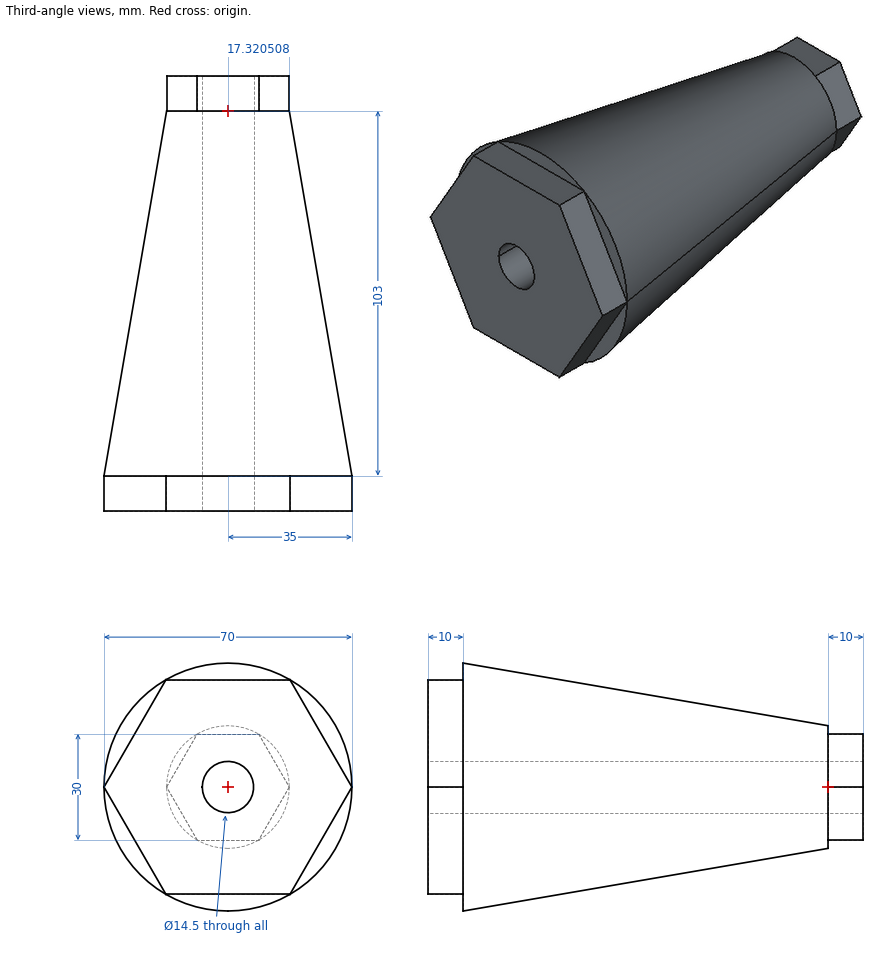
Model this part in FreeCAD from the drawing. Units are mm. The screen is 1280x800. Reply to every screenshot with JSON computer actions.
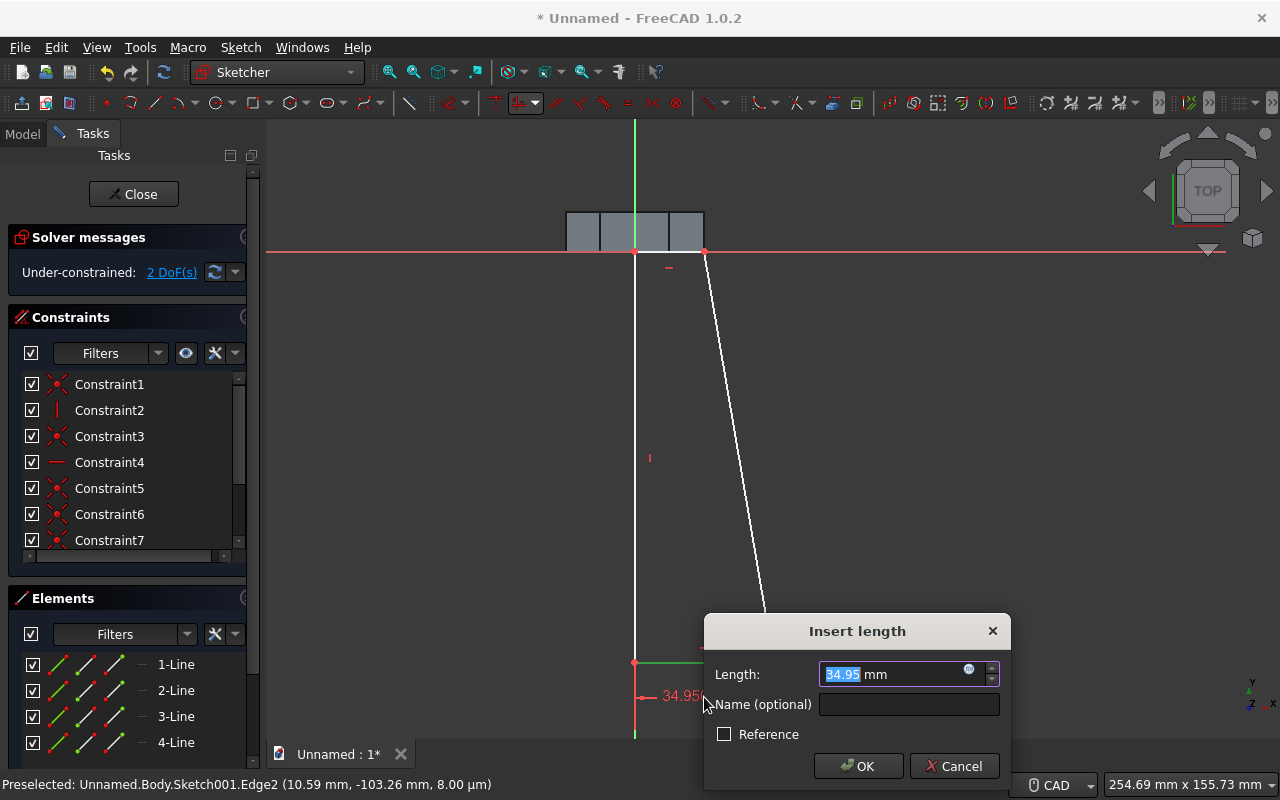
{"action": "type", "text": "35"}
{"action": "key", "text": "Return"}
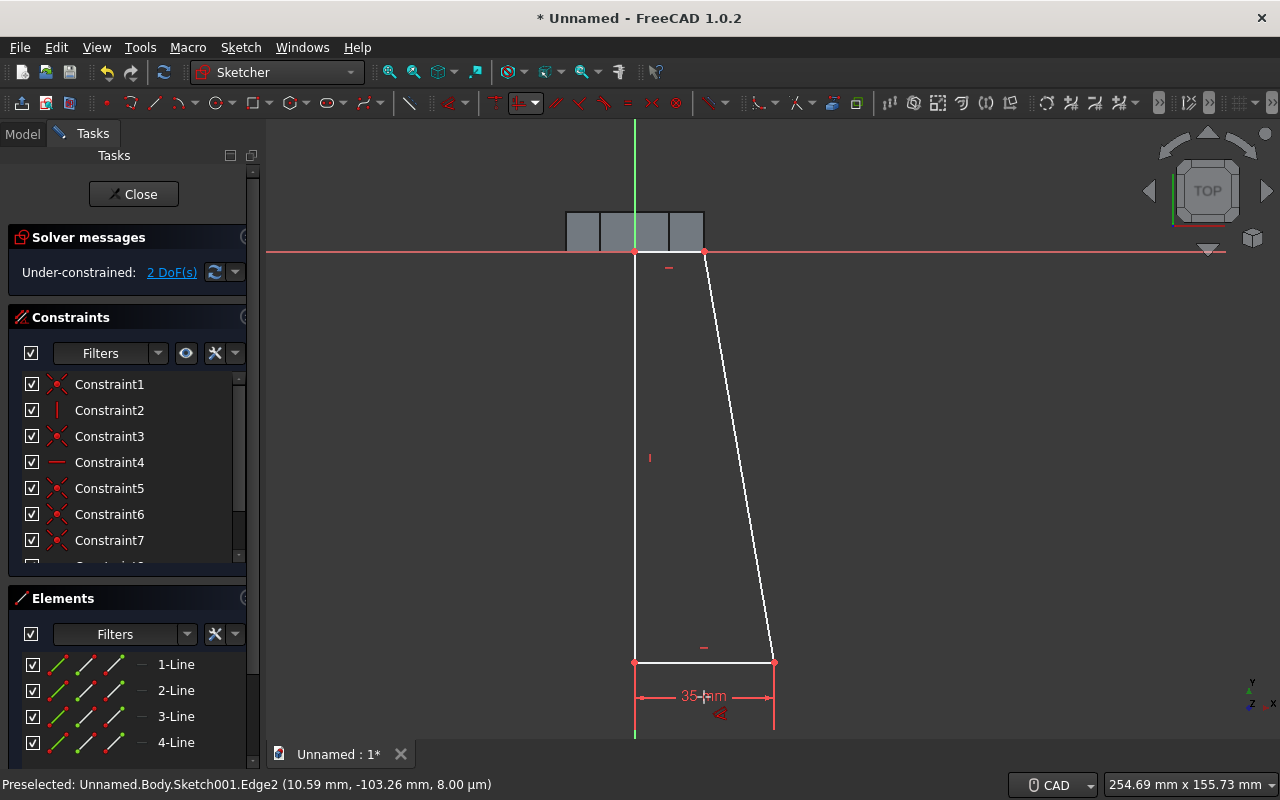
{"action": "left_click", "coordinate": [635, 375]}
{"action": "left_click", "coordinate": [601, 457]}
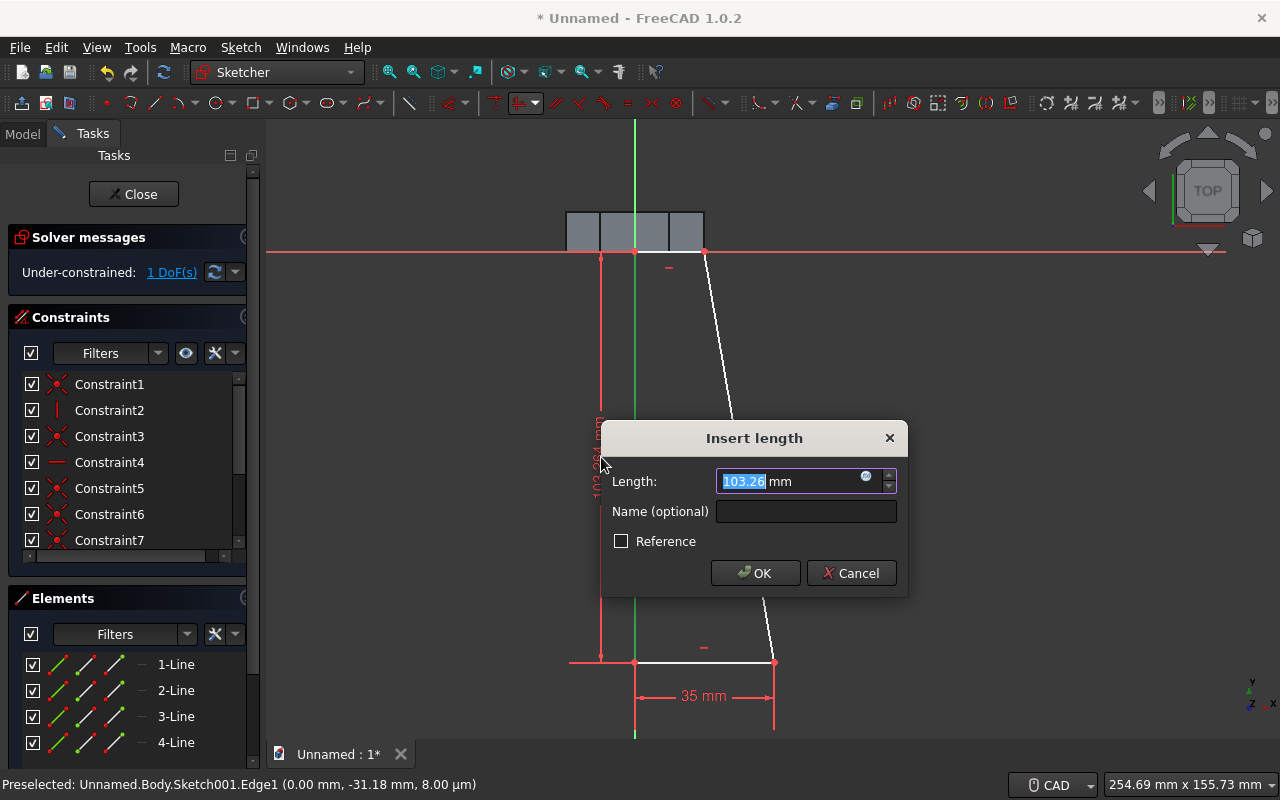
{"action": "type", "text": "103"}
{"action": "key", "text": "Return"}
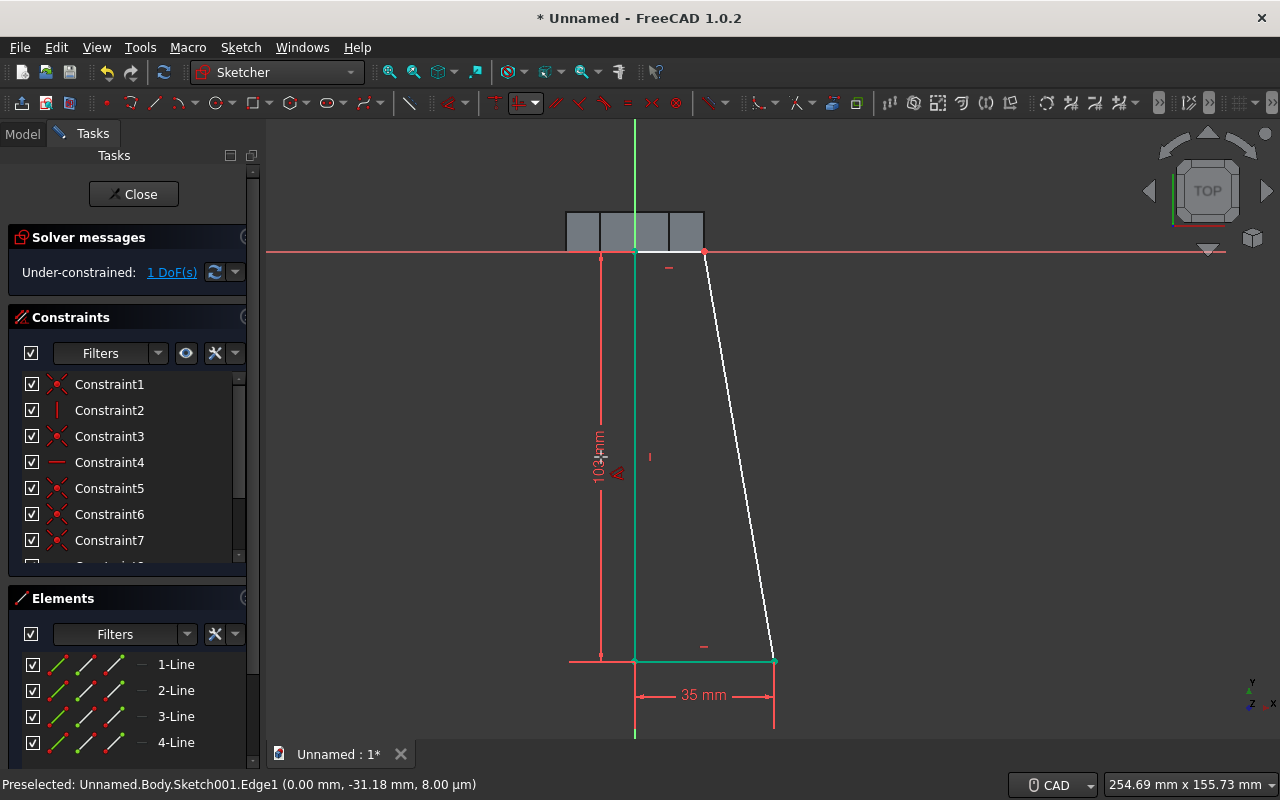
{"action": "left_click", "coordinate": [683, 252]}
{"action": "left_click", "coordinate": [669, 218]}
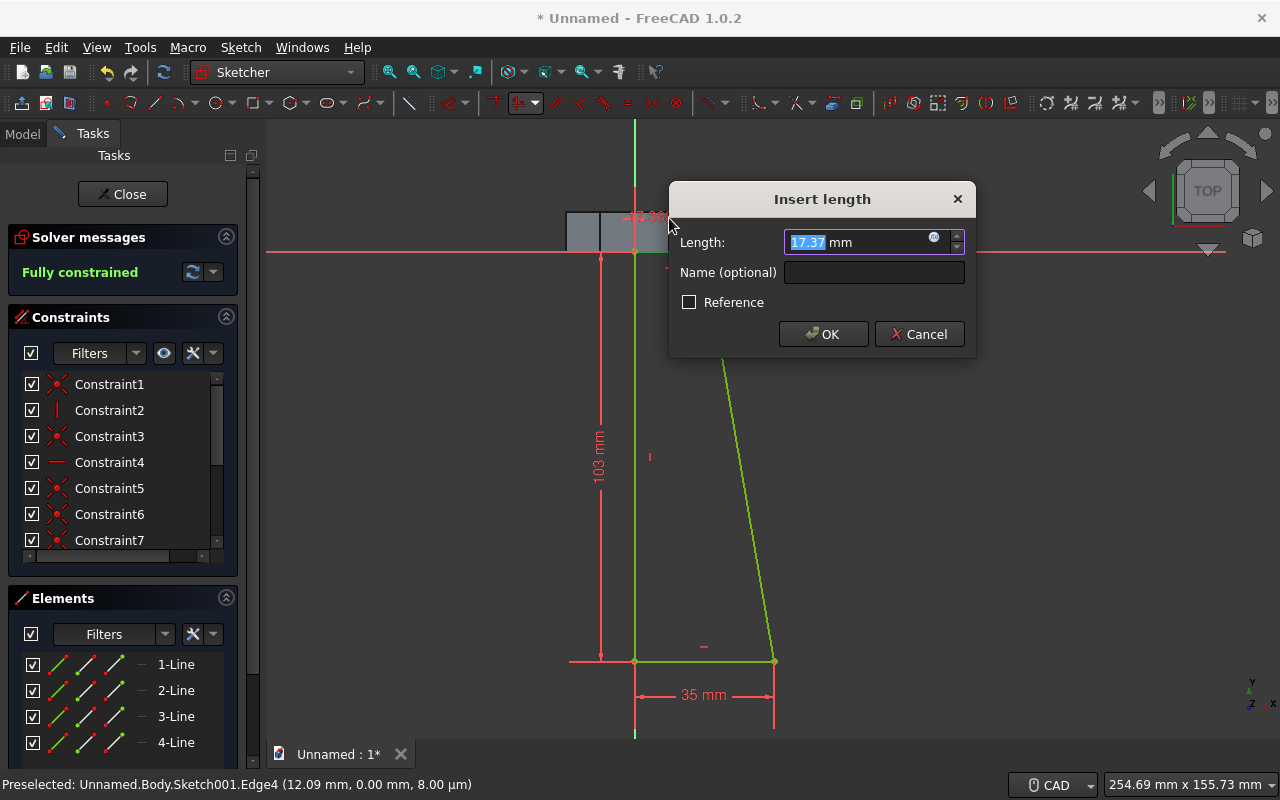
{"action": "type", "text": "17.320508"}
{"action": "key", "text": "Return"}
{"action": "key", "text": "Escape"}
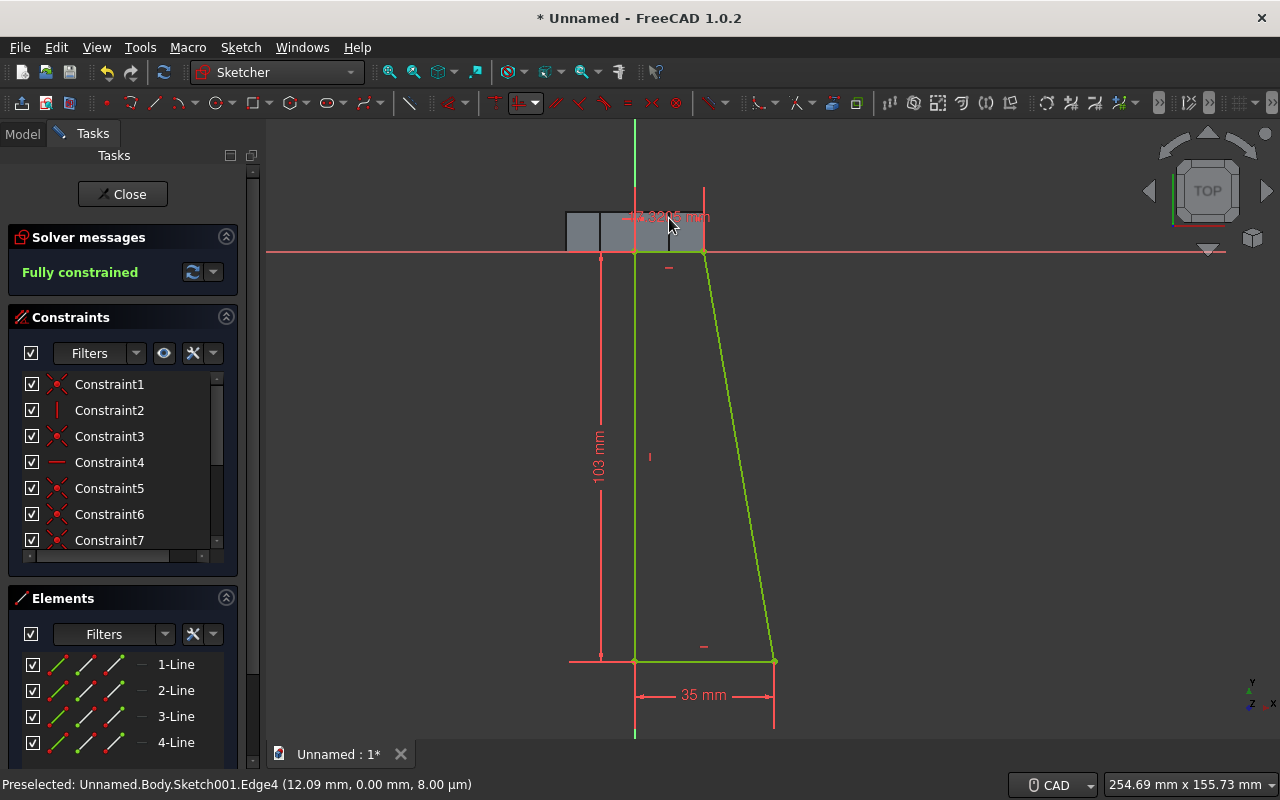
{"action": "left_click", "coordinate": [123, 194]}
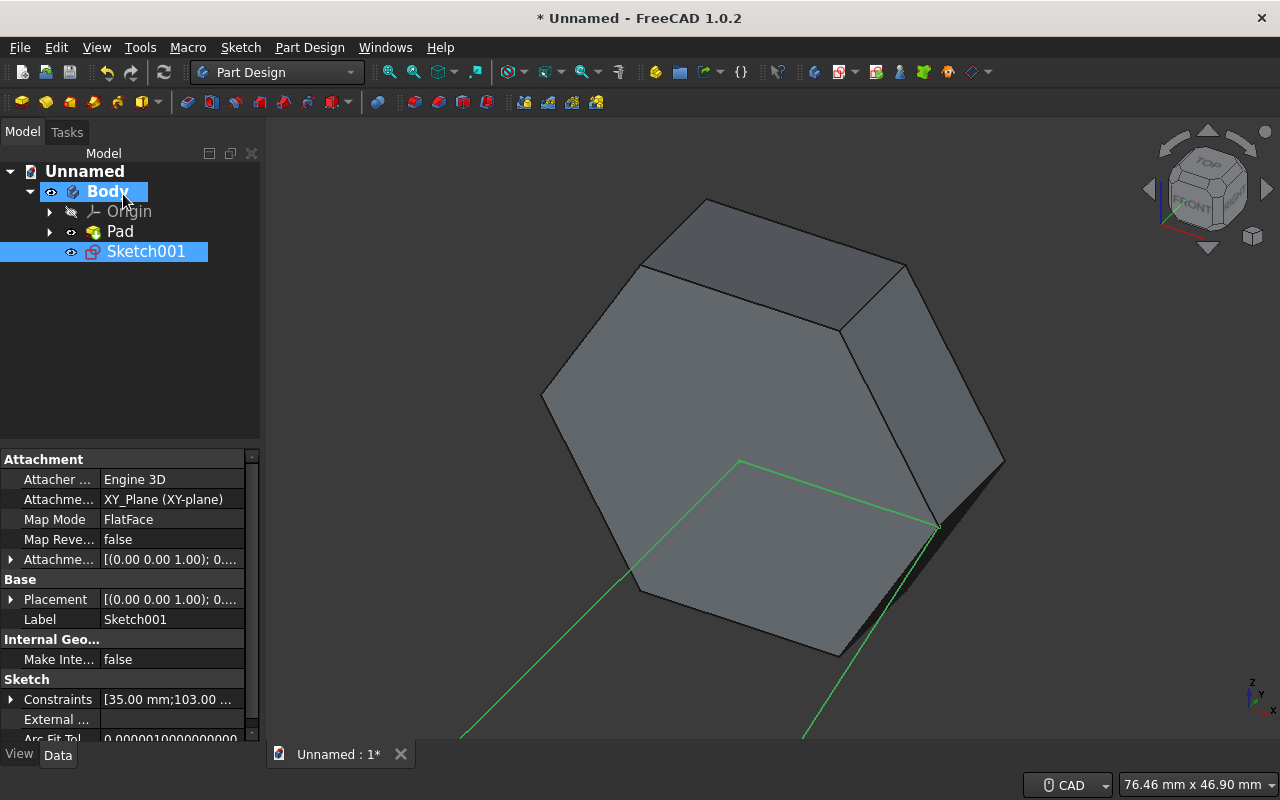
{"action": "left_click", "coordinate": [46, 102]}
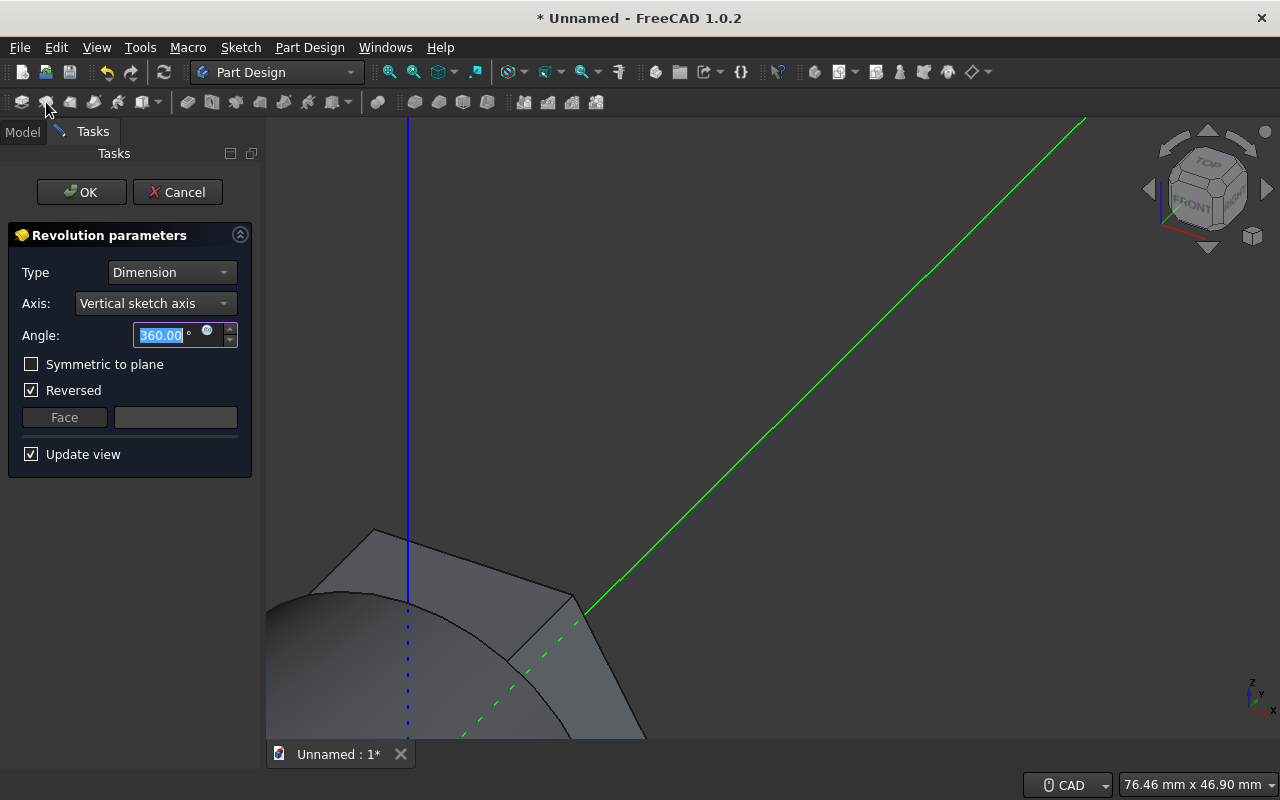
{"action": "left_click", "coordinate": [82, 192]}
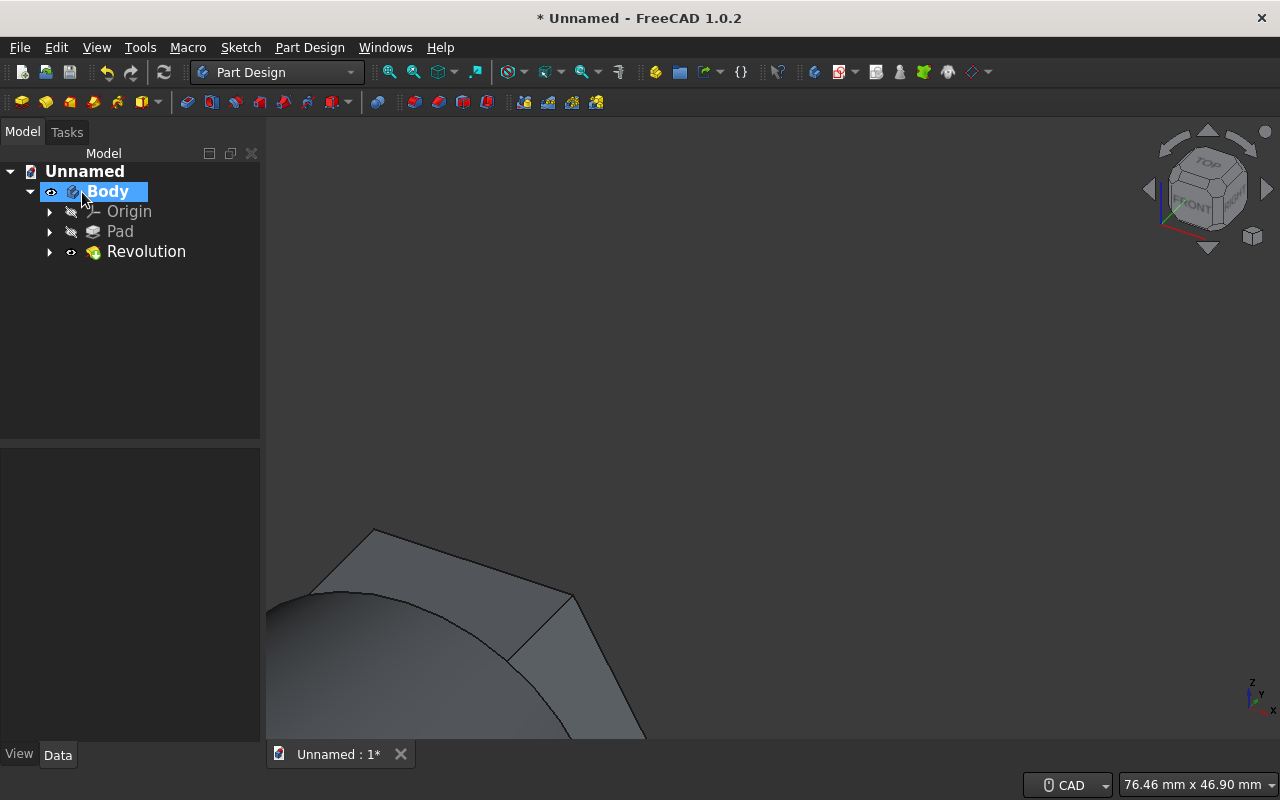
{"action": "key", "text": "v f"}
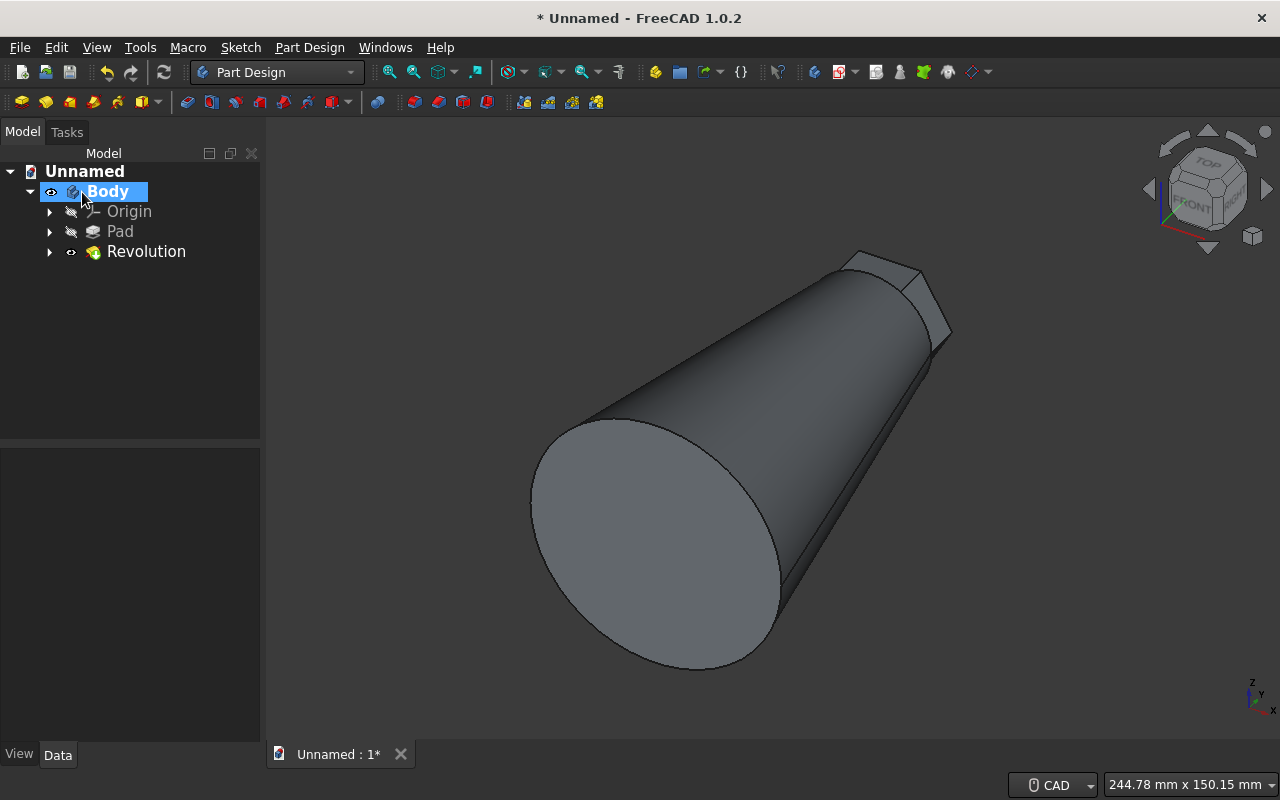
{"action": "left_click", "coordinate": [656, 543]}